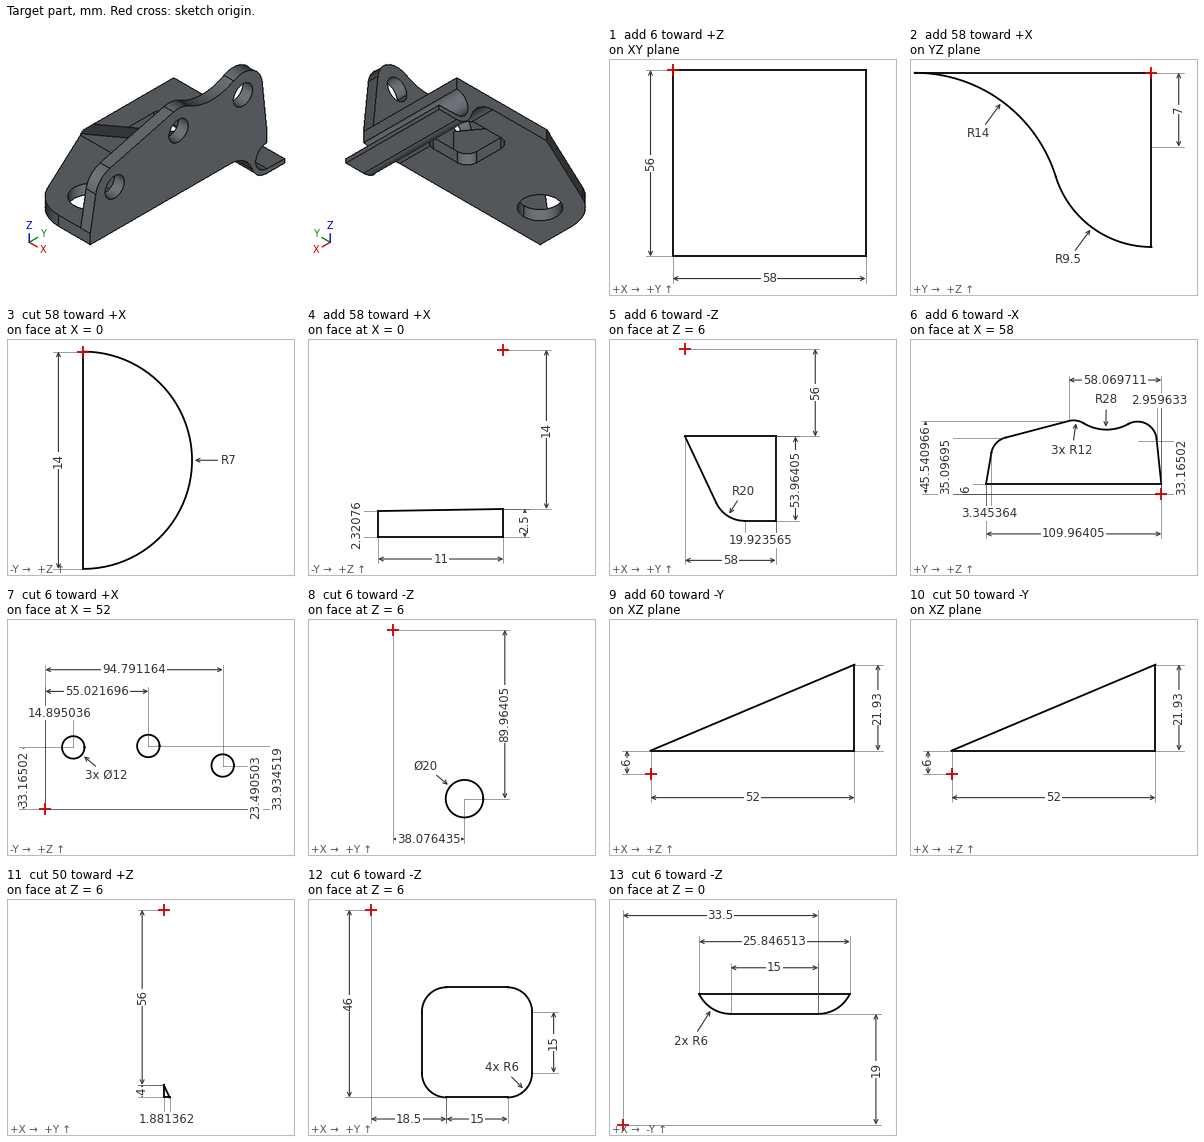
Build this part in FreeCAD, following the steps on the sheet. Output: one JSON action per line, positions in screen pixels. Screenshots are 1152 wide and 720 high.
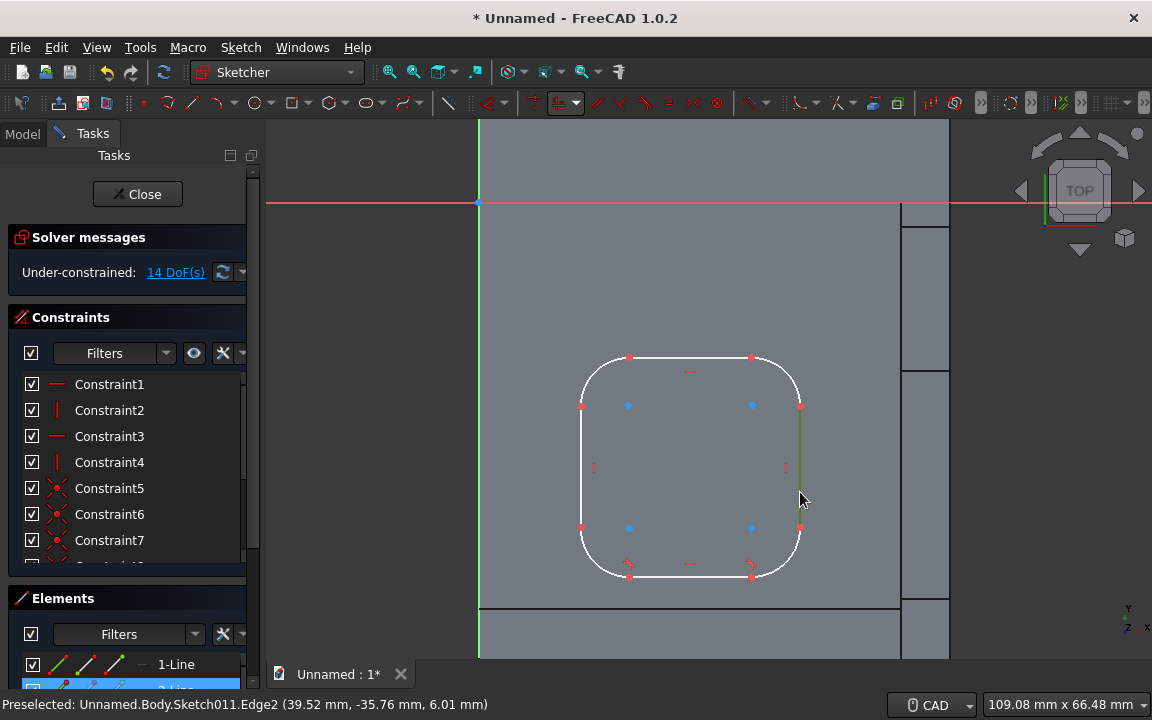
{"action": "left_click", "coordinate": [773, 572]}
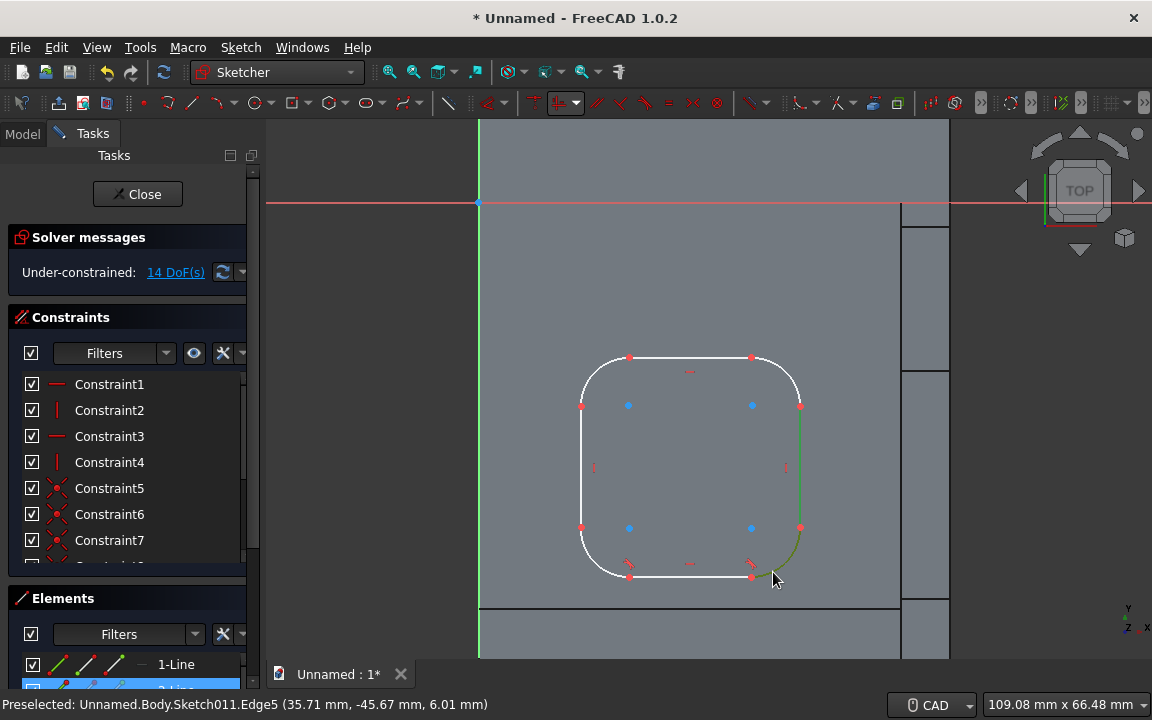
{"action": "left_click", "coordinate": [646, 104]}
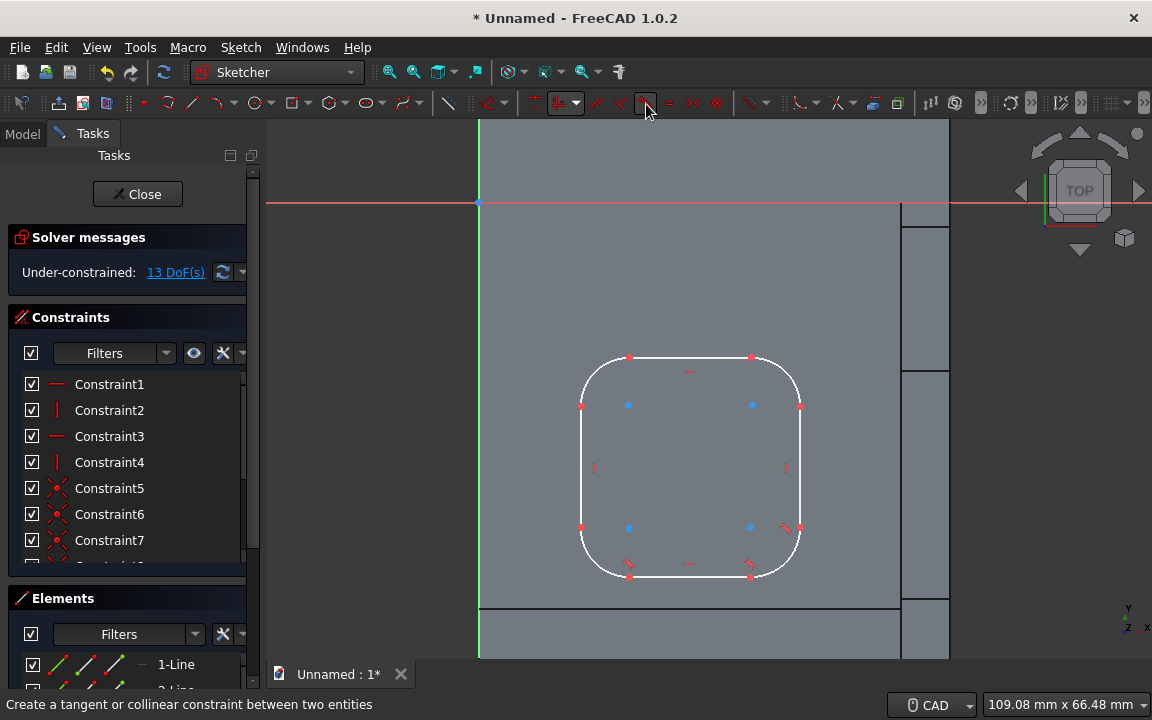
{"action": "left_click", "coordinate": [800, 492]}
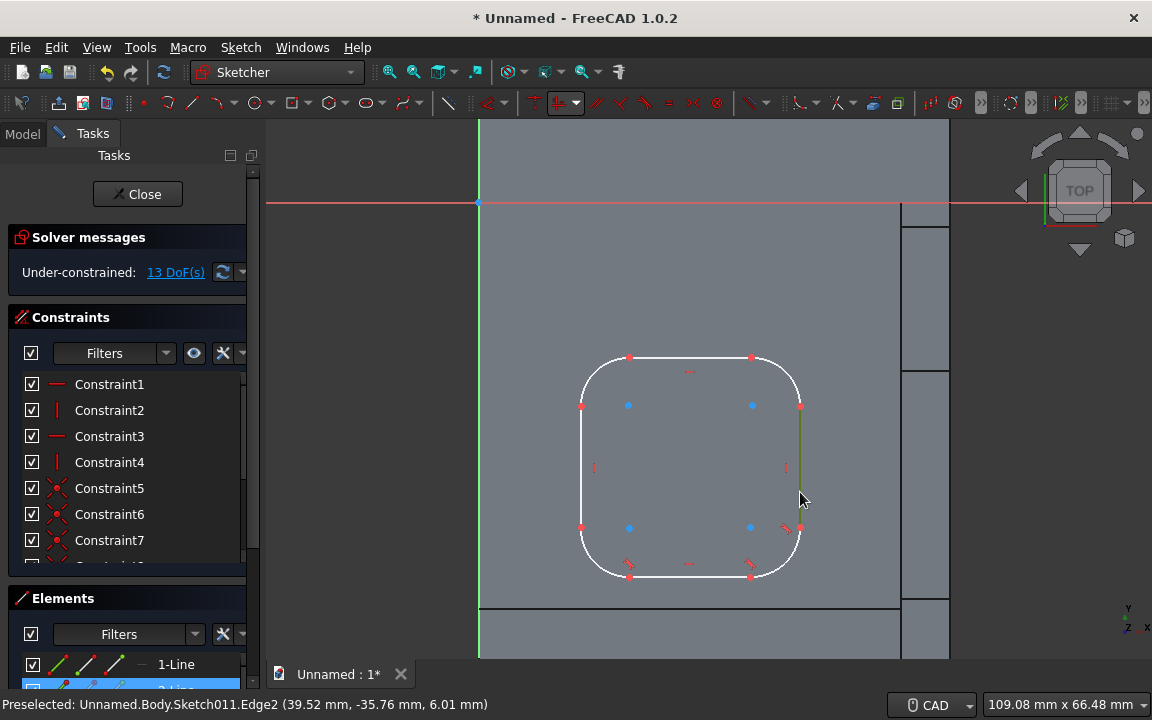
{"action": "left_click", "coordinate": [795, 385]}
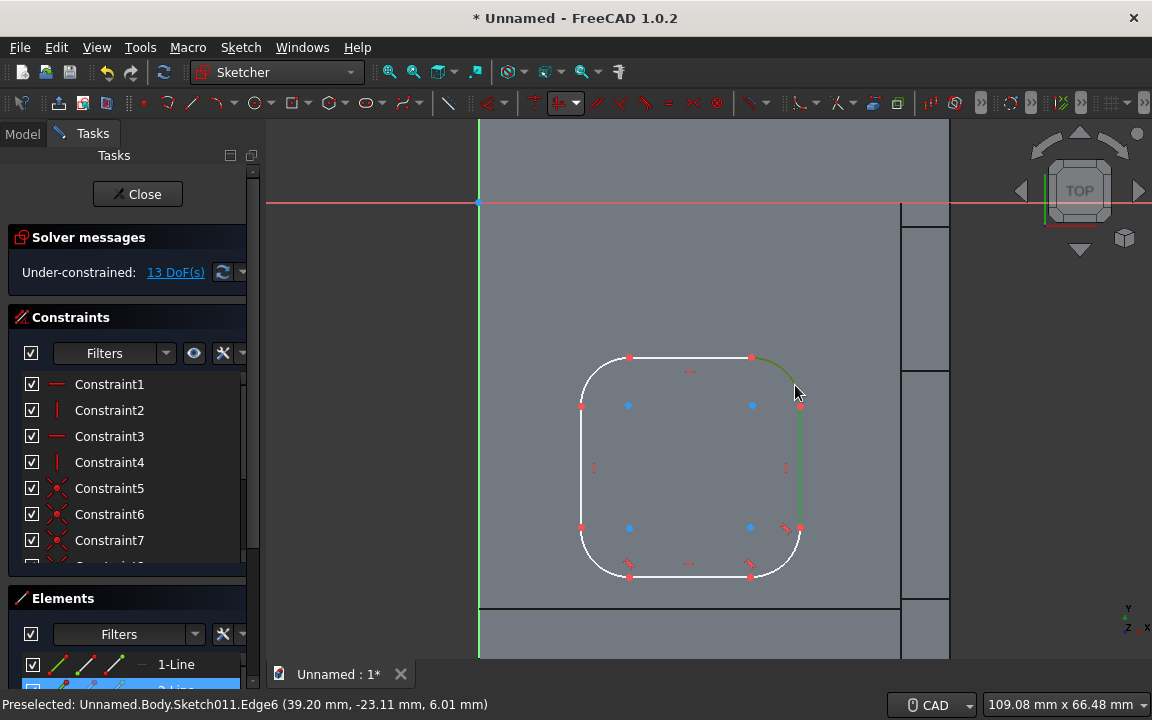
{"action": "left_click", "coordinate": [646, 104]}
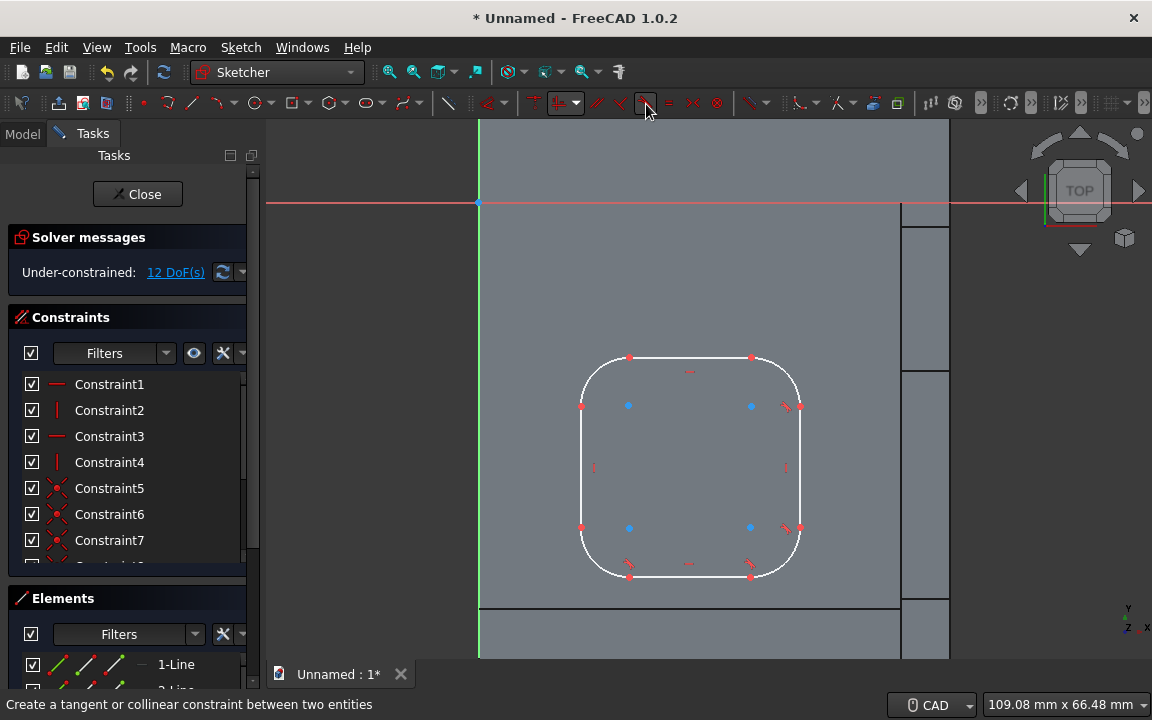
{"action": "left_click", "coordinate": [714, 358]}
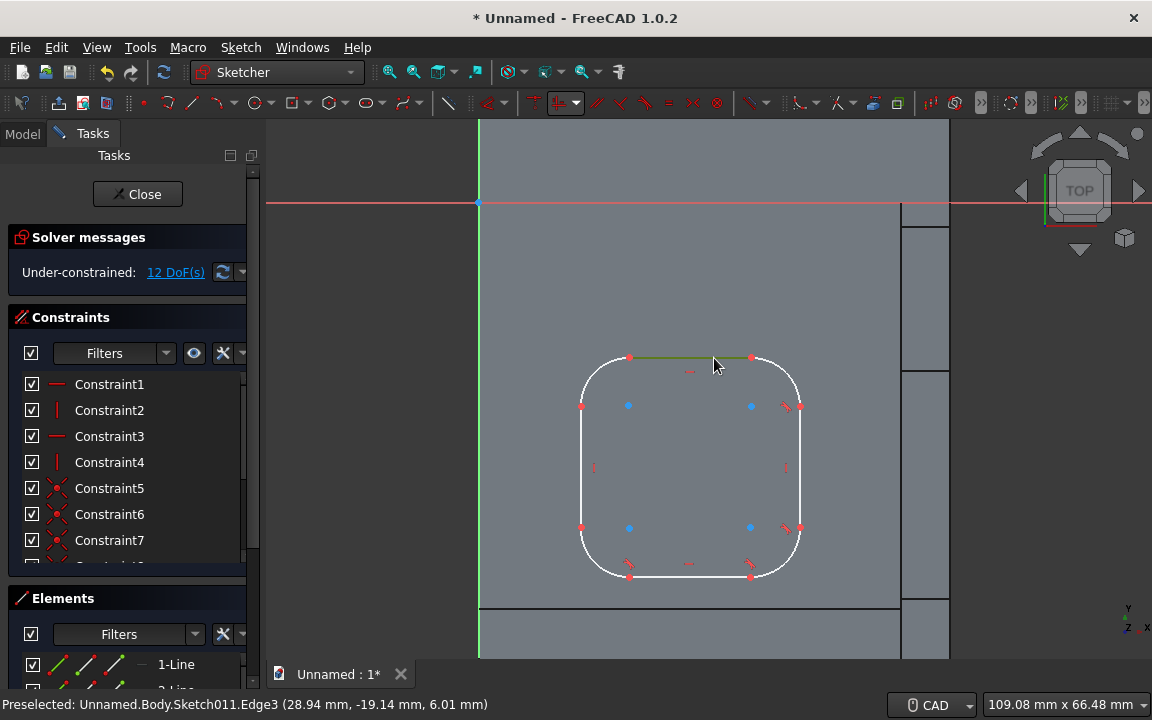
{"action": "left_click", "coordinate": [795, 385]}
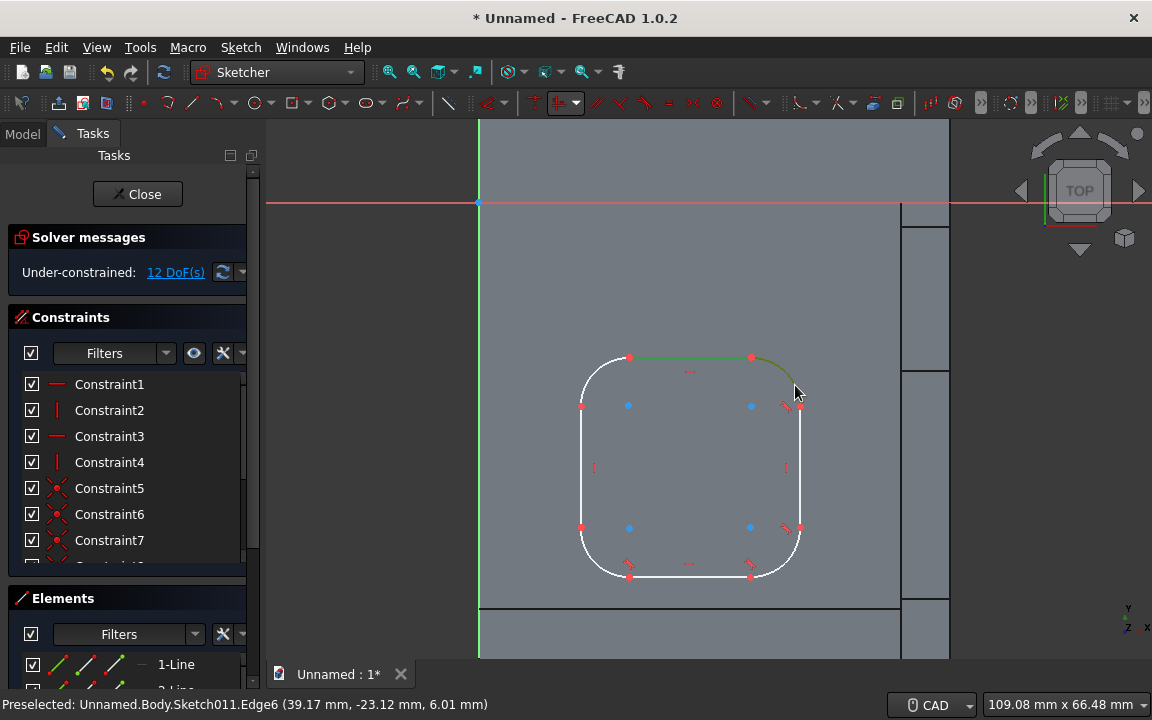
{"action": "key", "text": "t"}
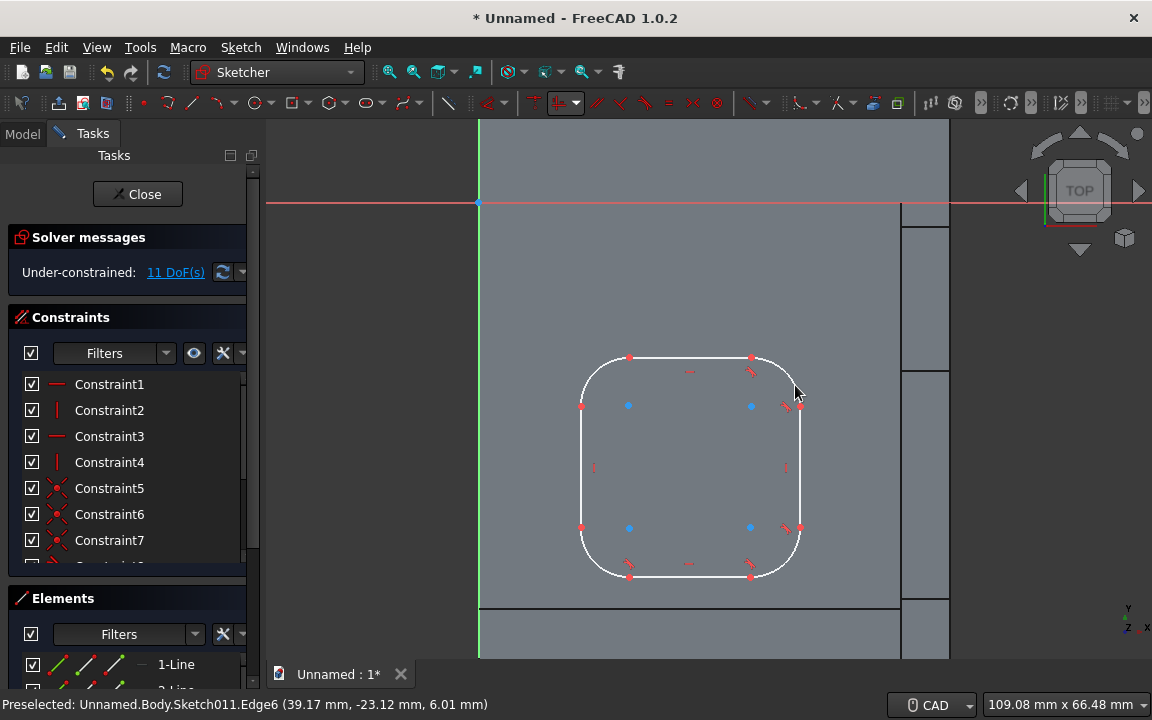
{"action": "left_click", "coordinate": [714, 358]}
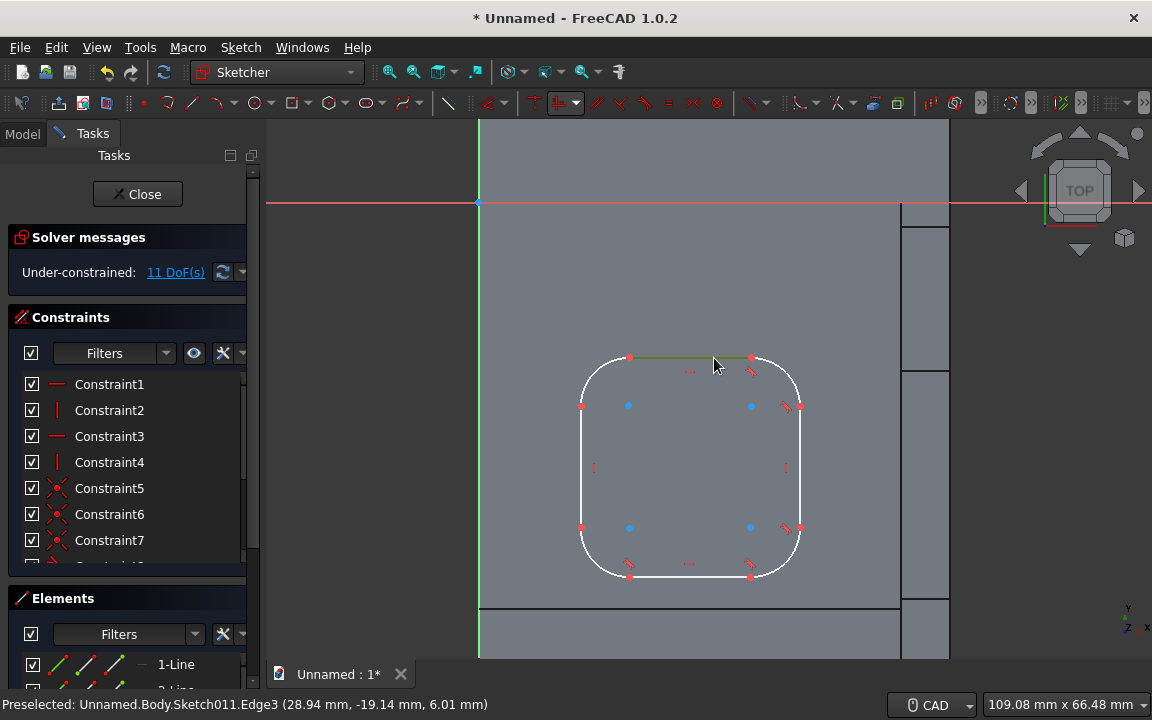
{"action": "left_click", "coordinate": [607, 363]}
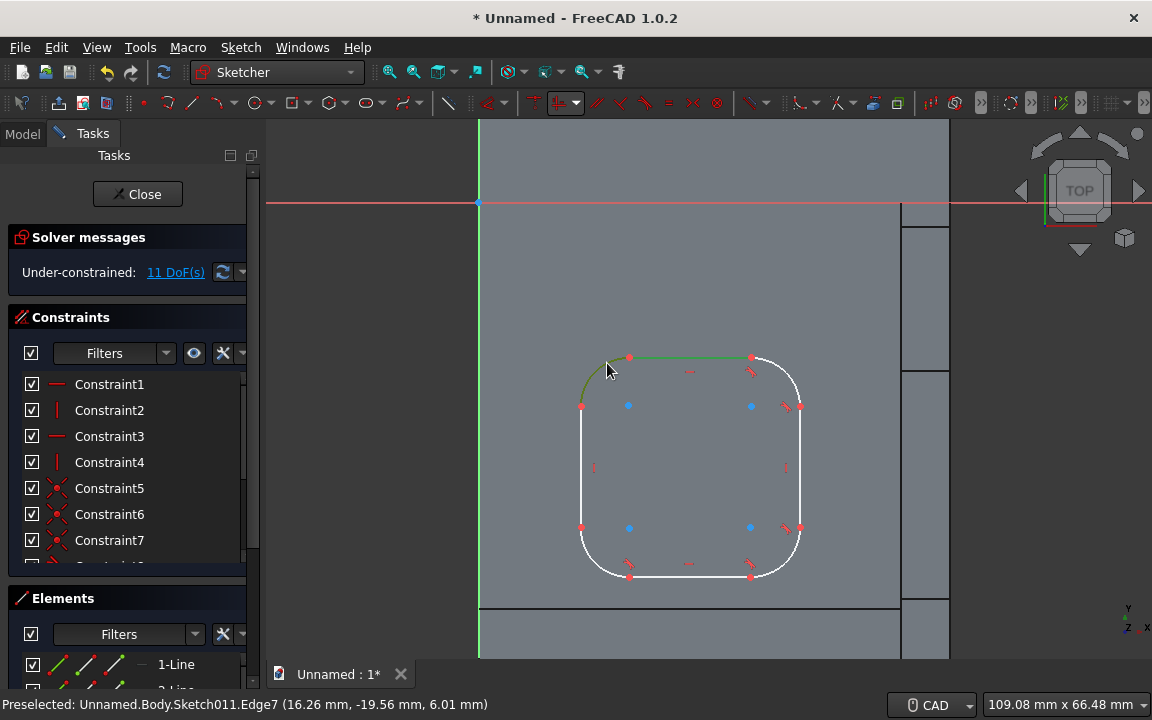
{"action": "left_click", "coordinate": [646, 104]}